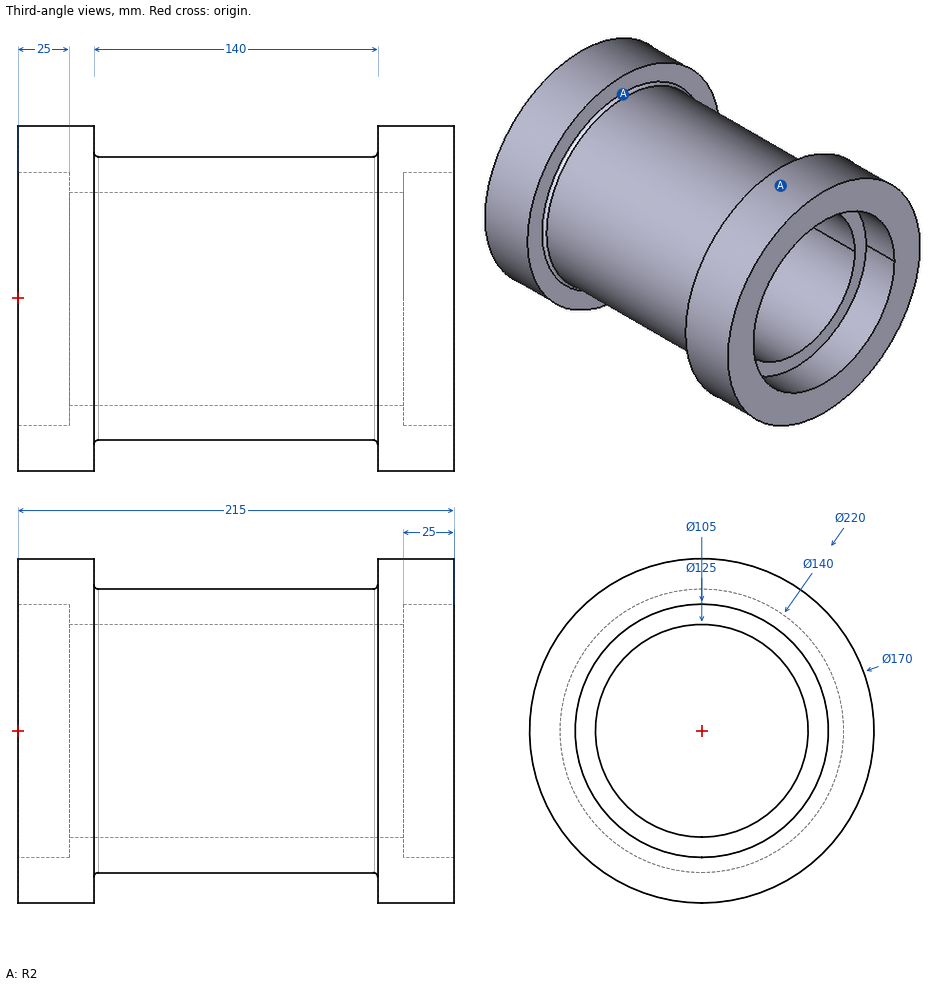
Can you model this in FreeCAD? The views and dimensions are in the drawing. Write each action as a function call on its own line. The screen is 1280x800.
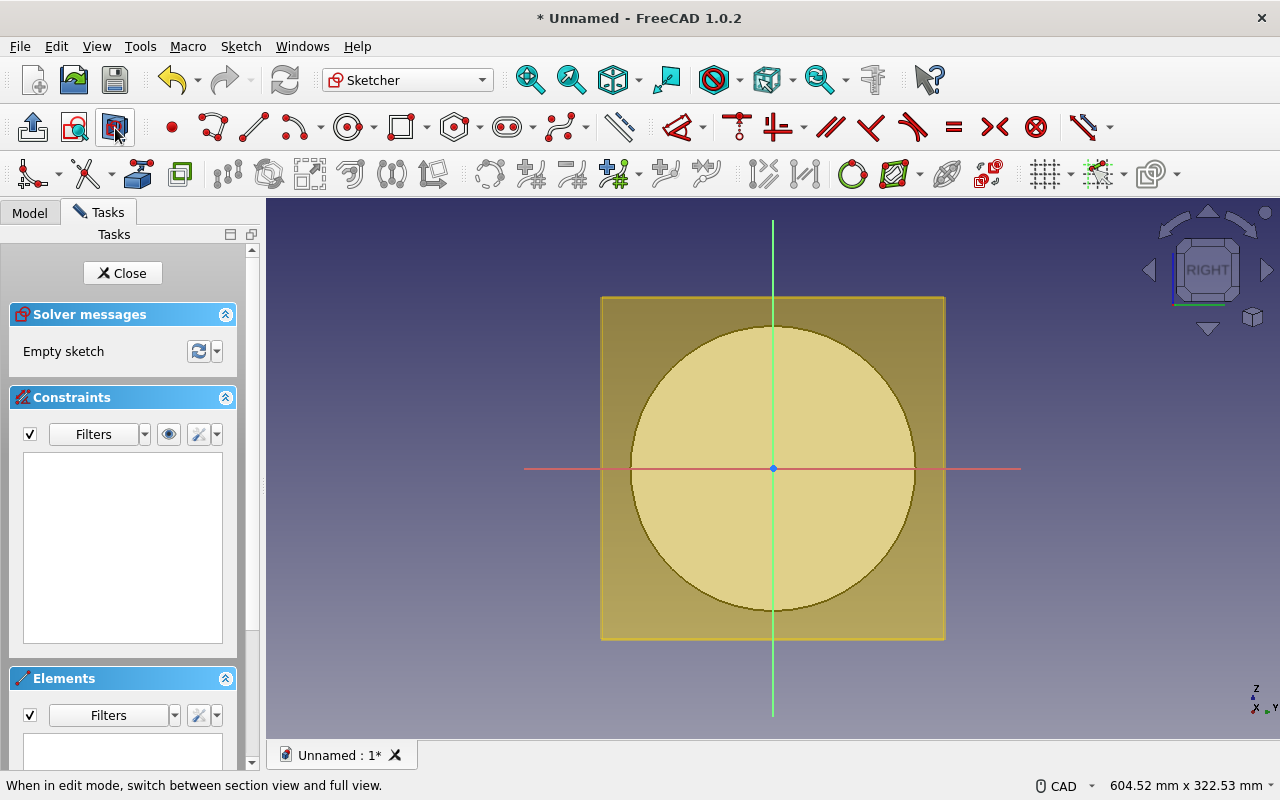
scroll(912, 469, up, 2)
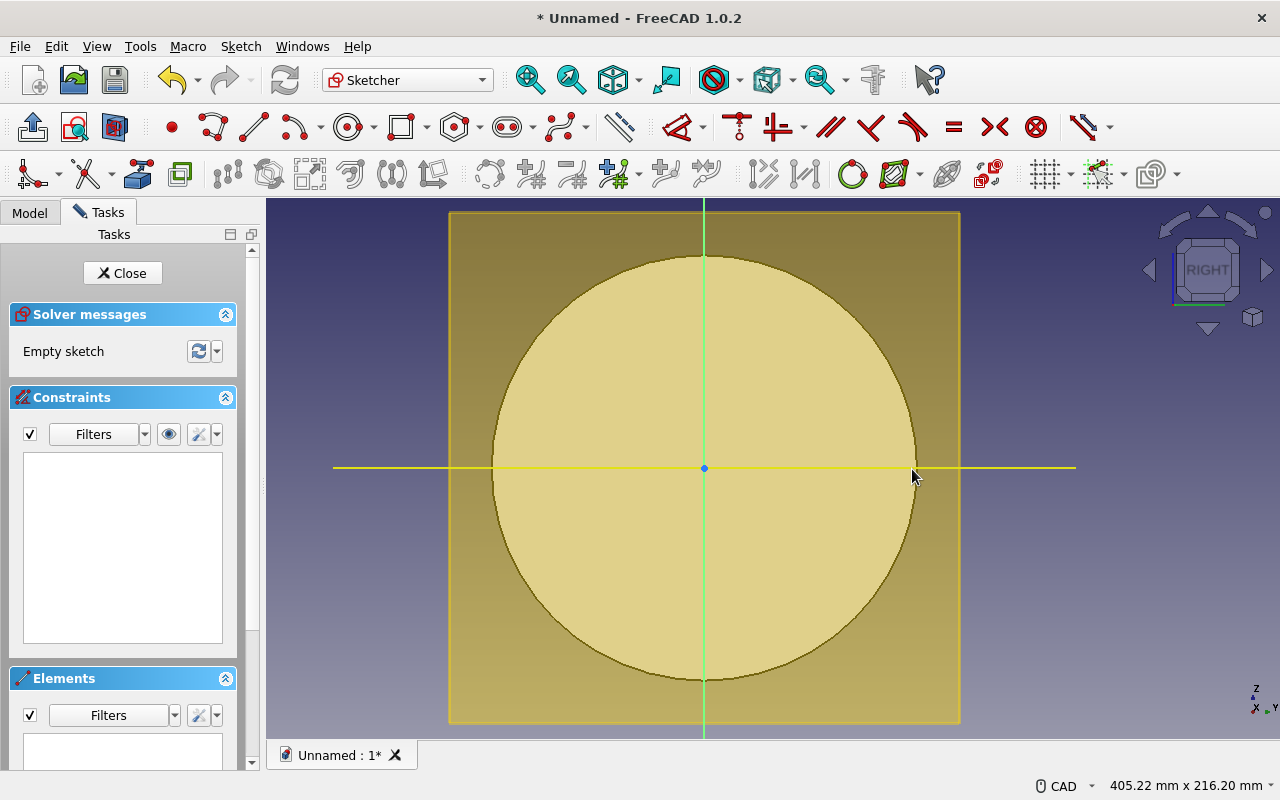
key(g)
key(c)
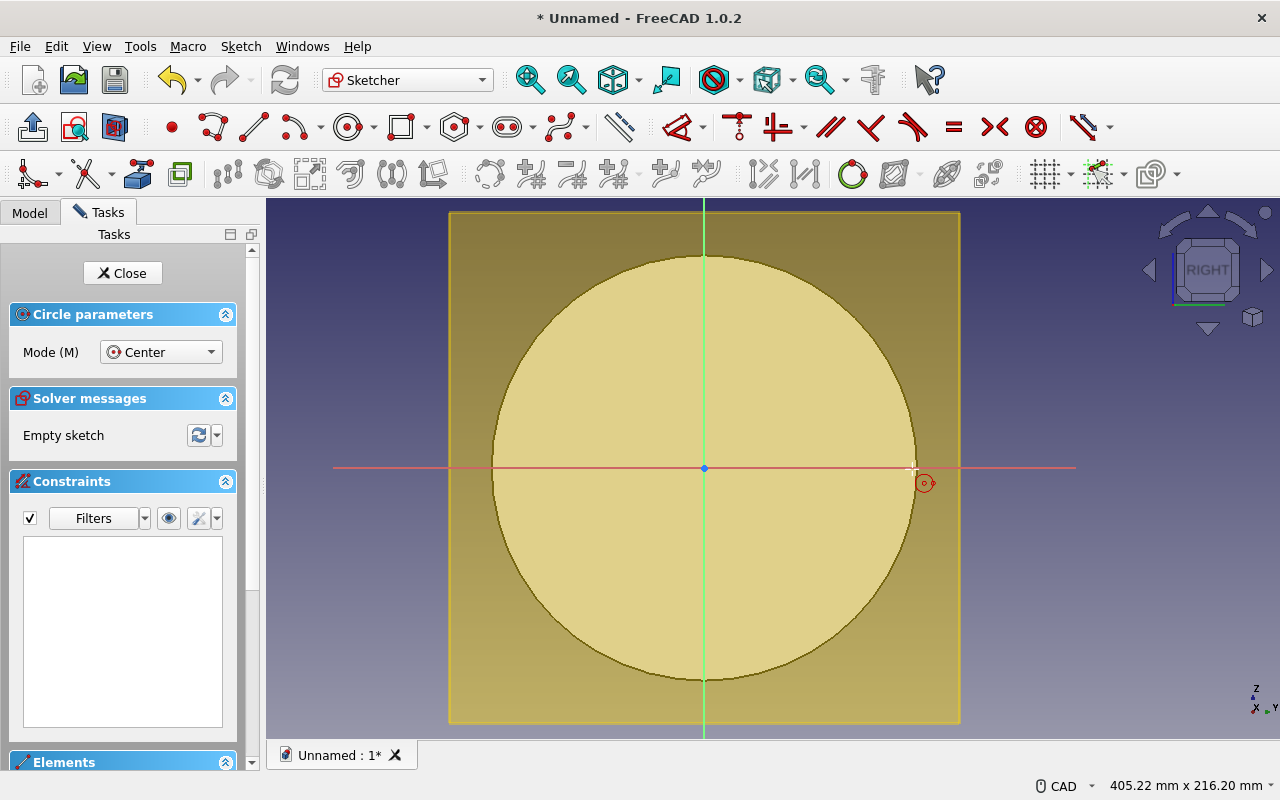
click(704, 468)
move(815, 357)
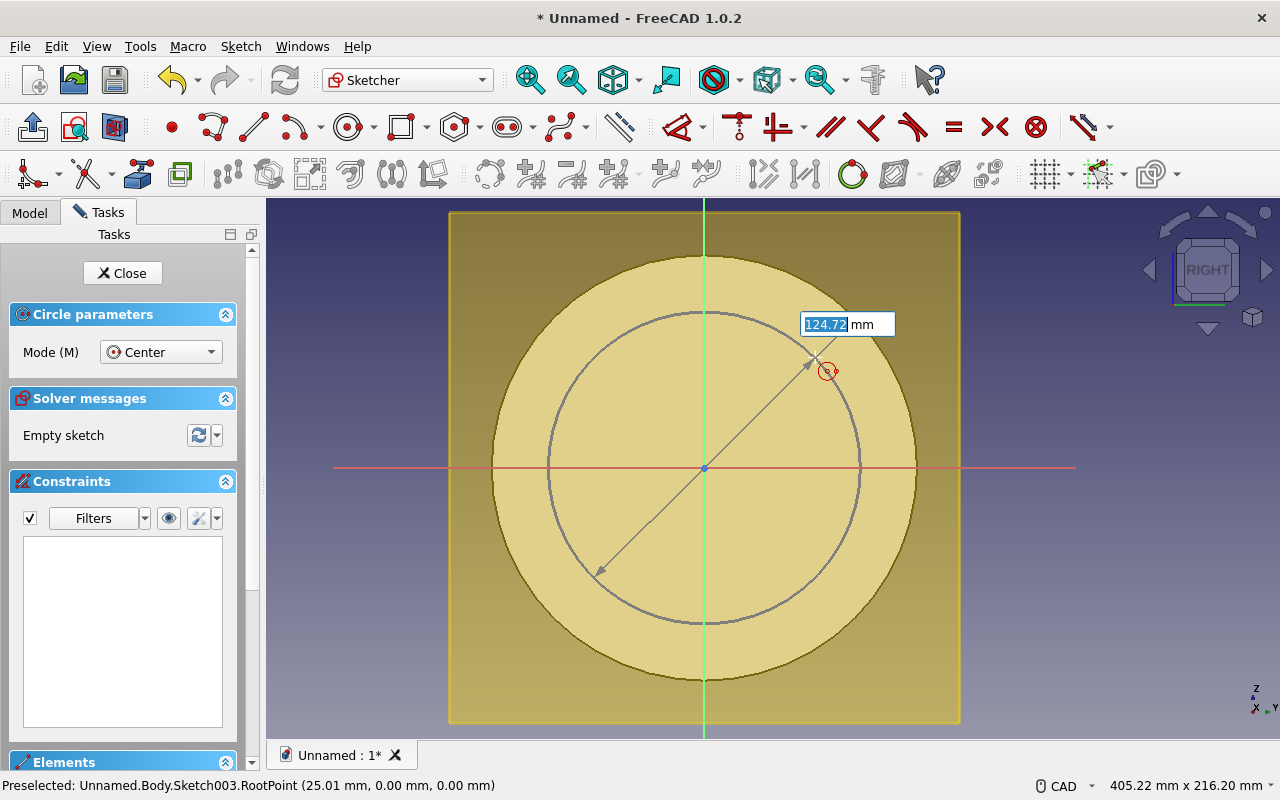
text(125)
key(Return)
key(Escape)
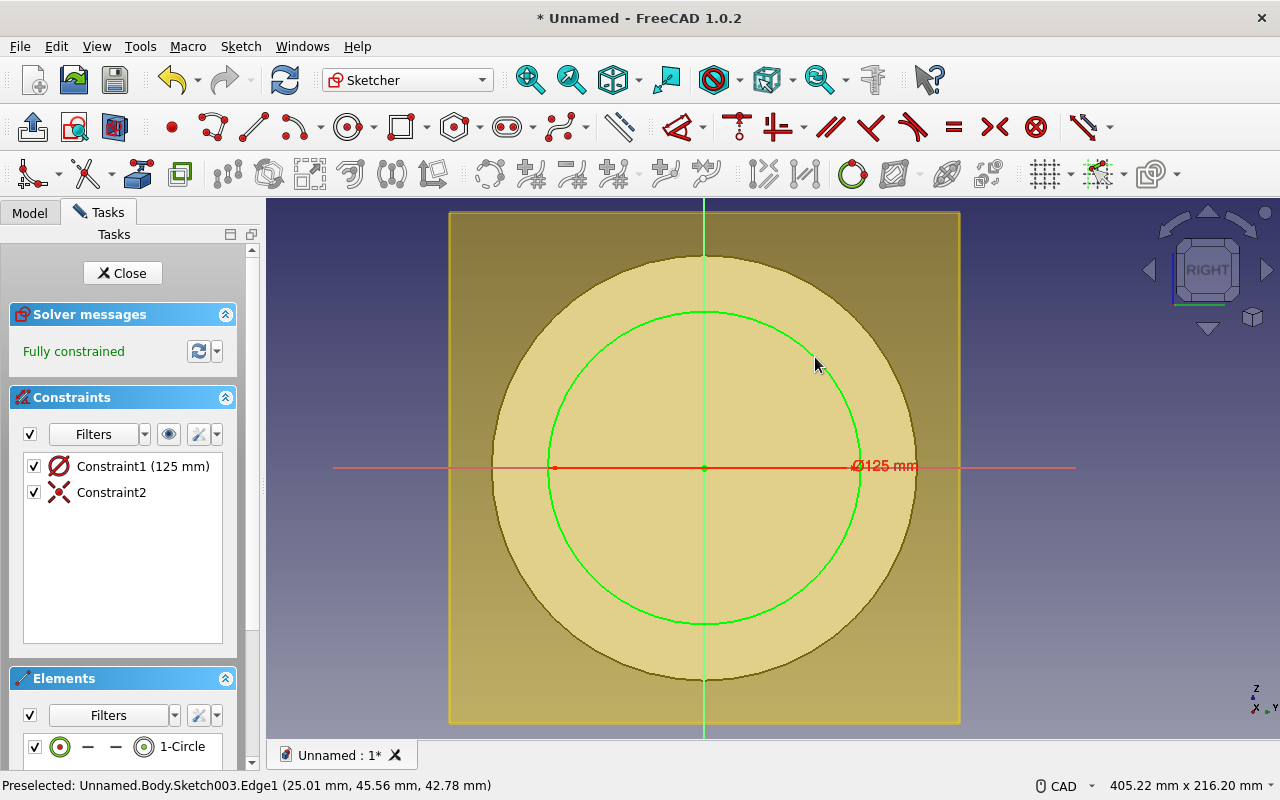
click(123, 273)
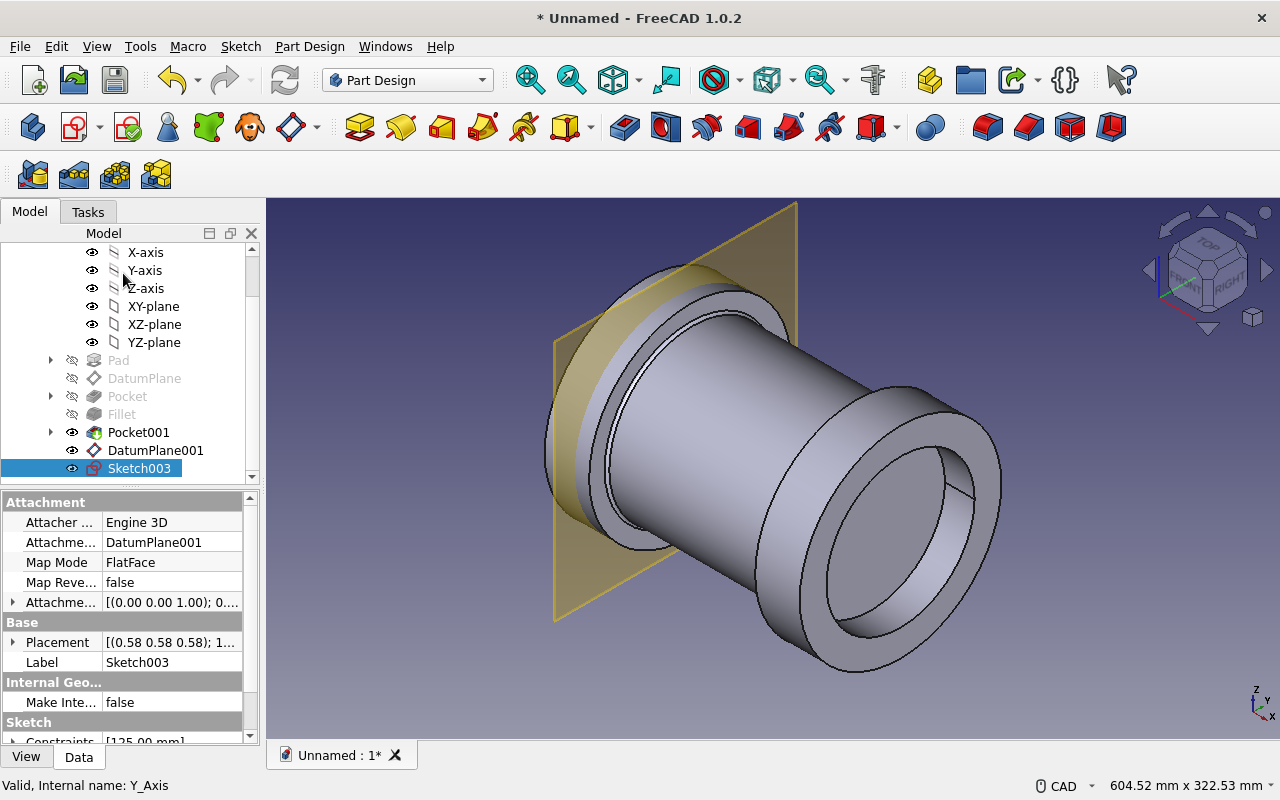
click(625, 128)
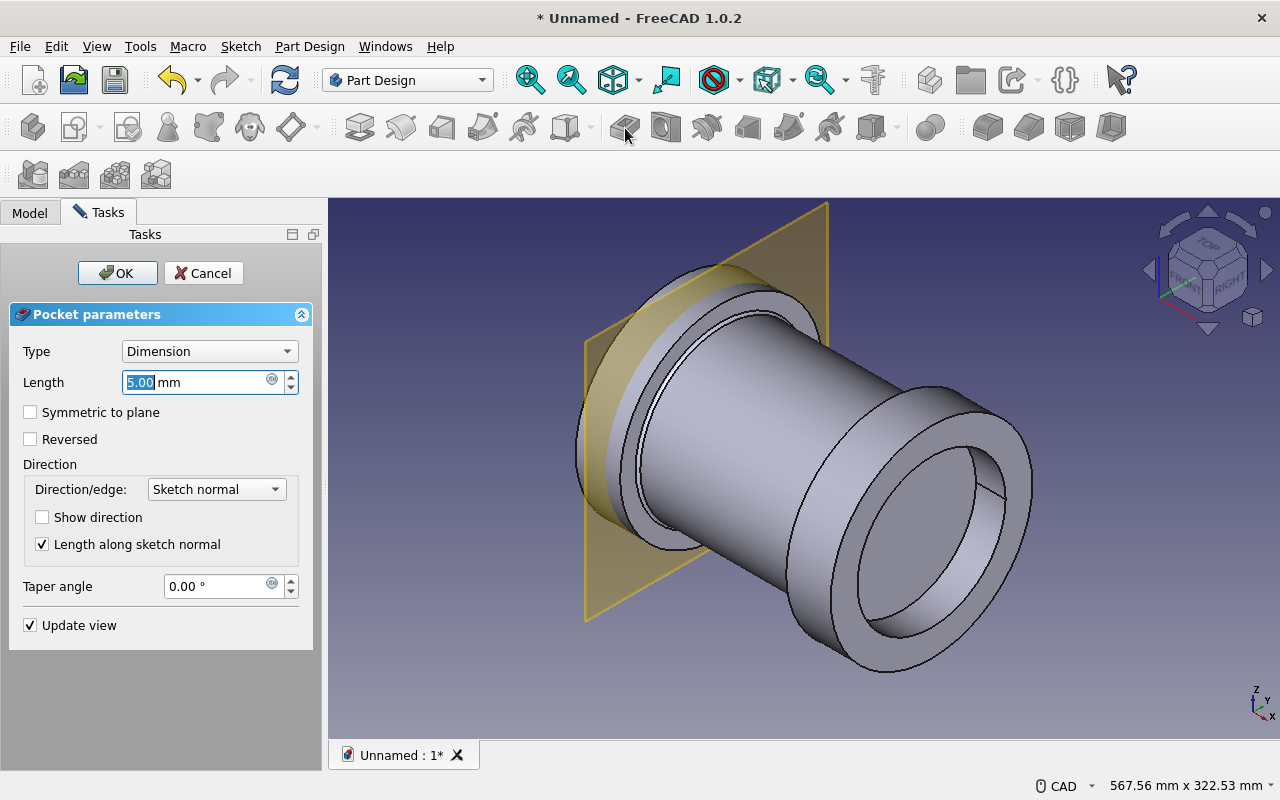
text(25)
key(Tab)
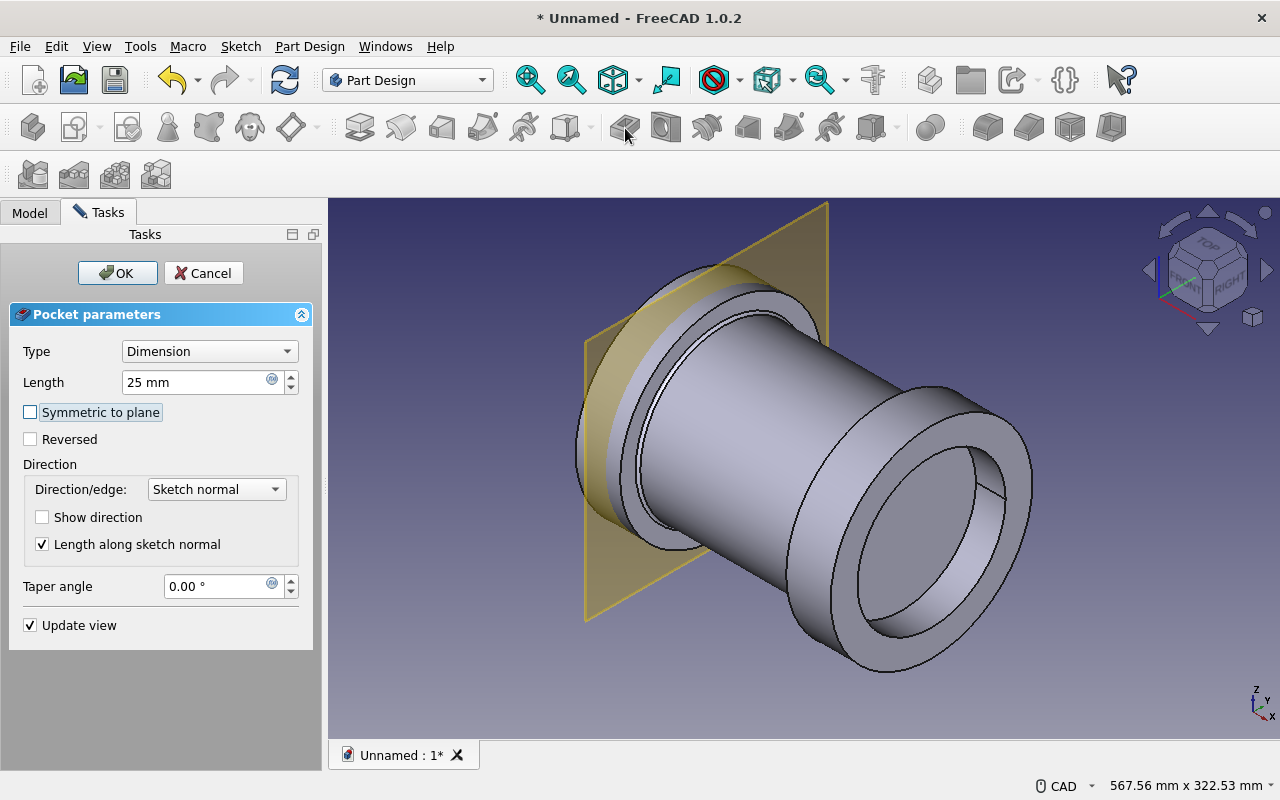
click(118, 273)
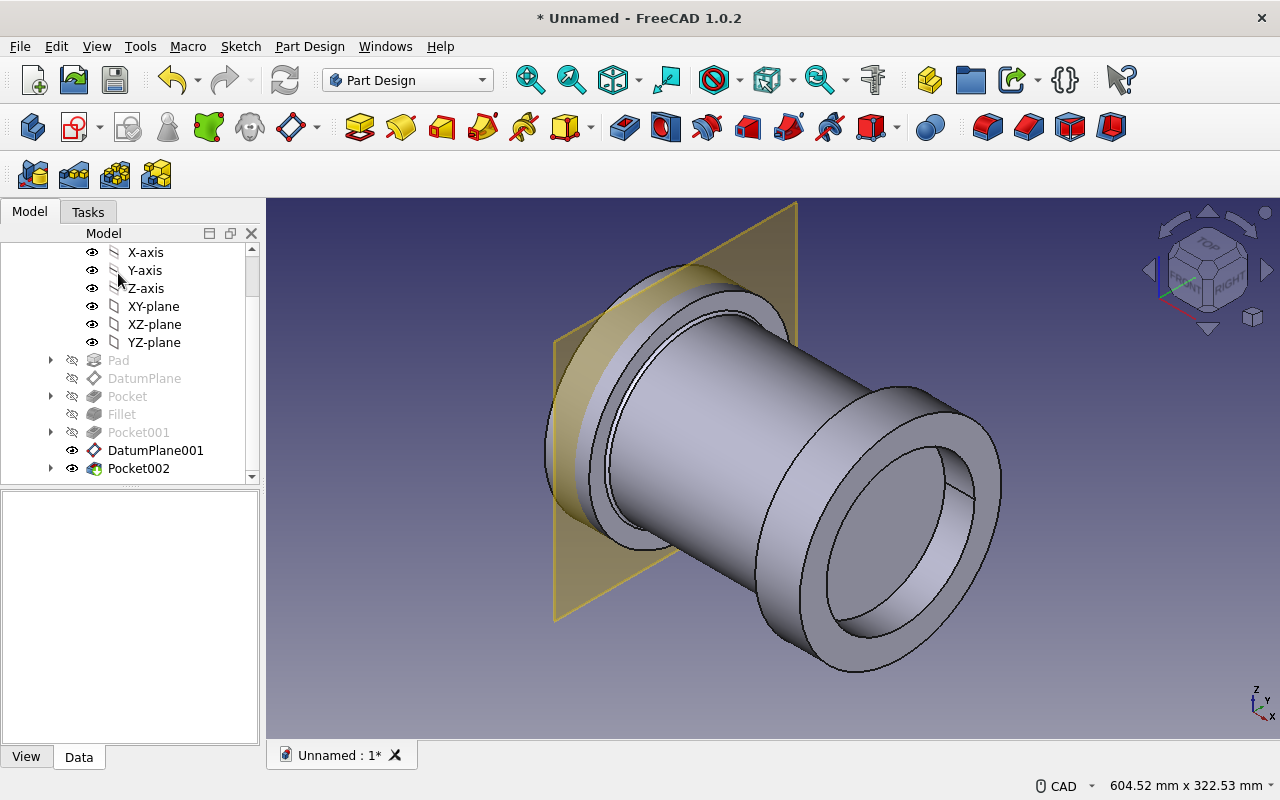
click(117, 450)
key(space)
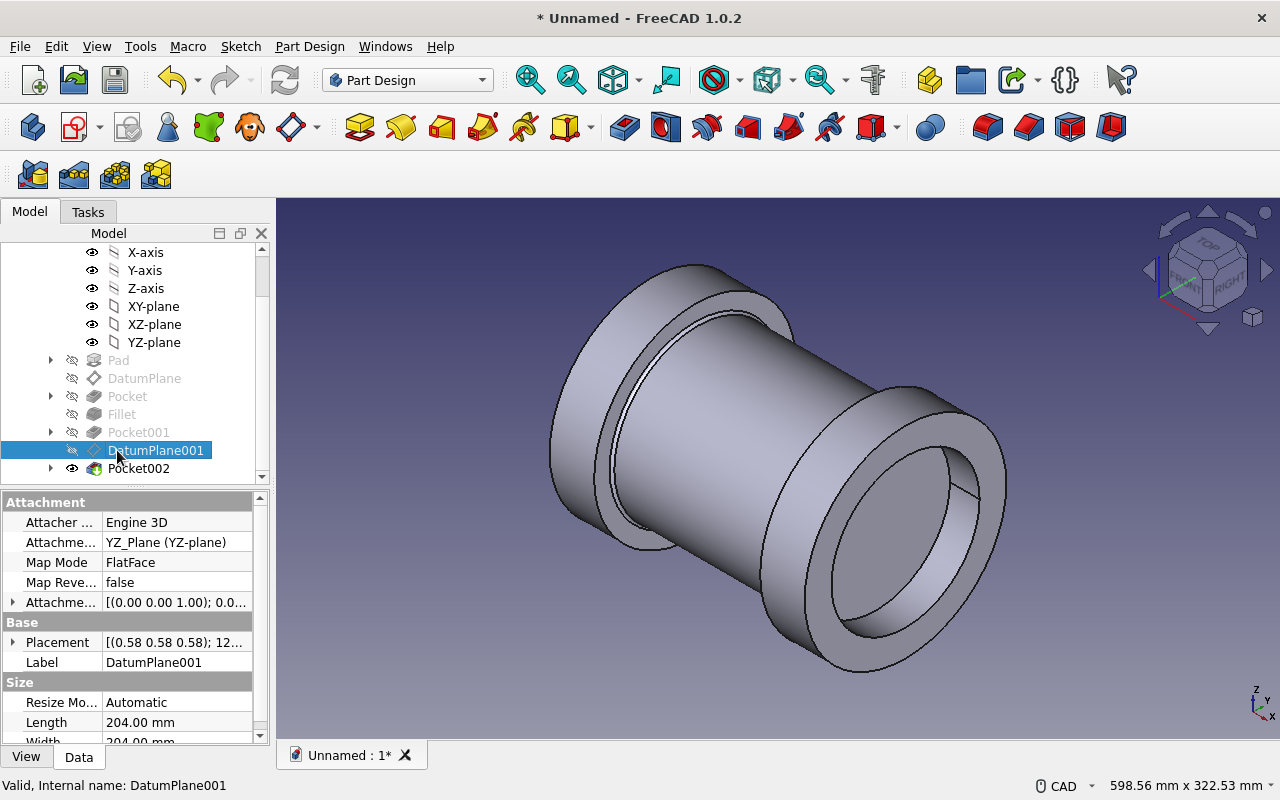
click(876, 524)